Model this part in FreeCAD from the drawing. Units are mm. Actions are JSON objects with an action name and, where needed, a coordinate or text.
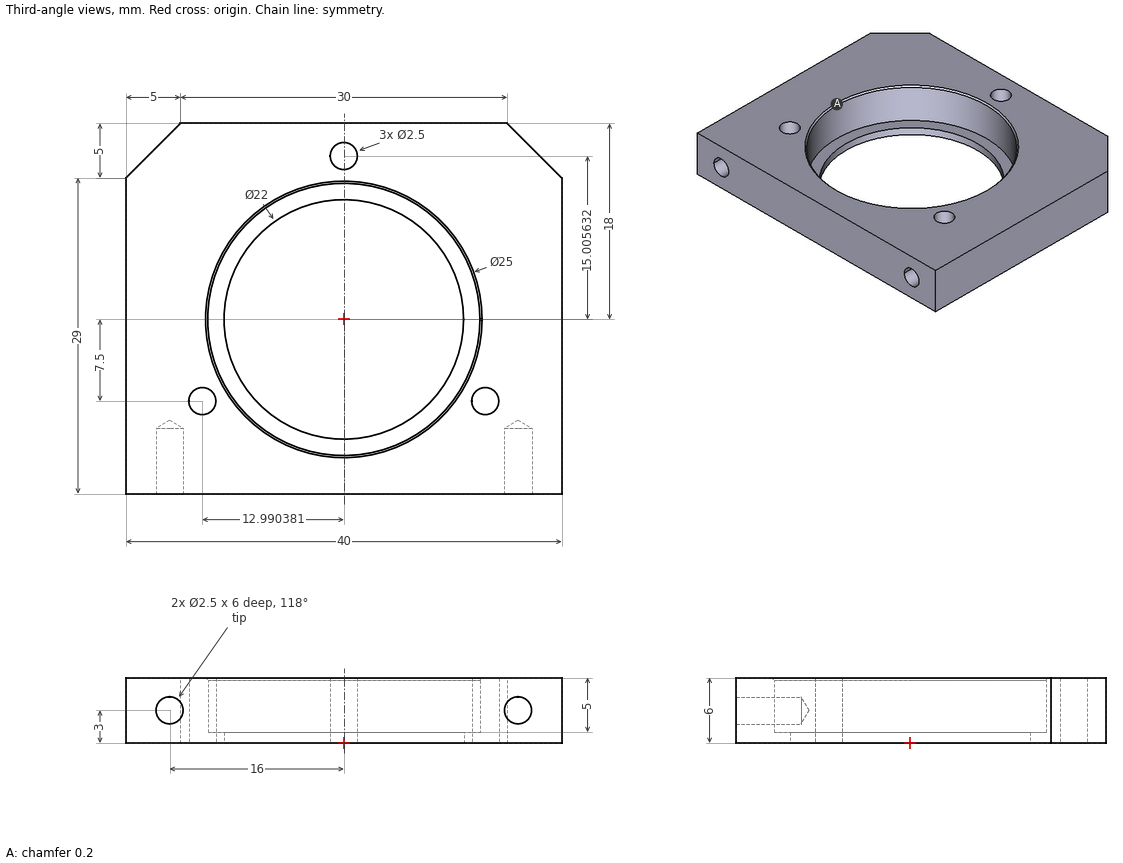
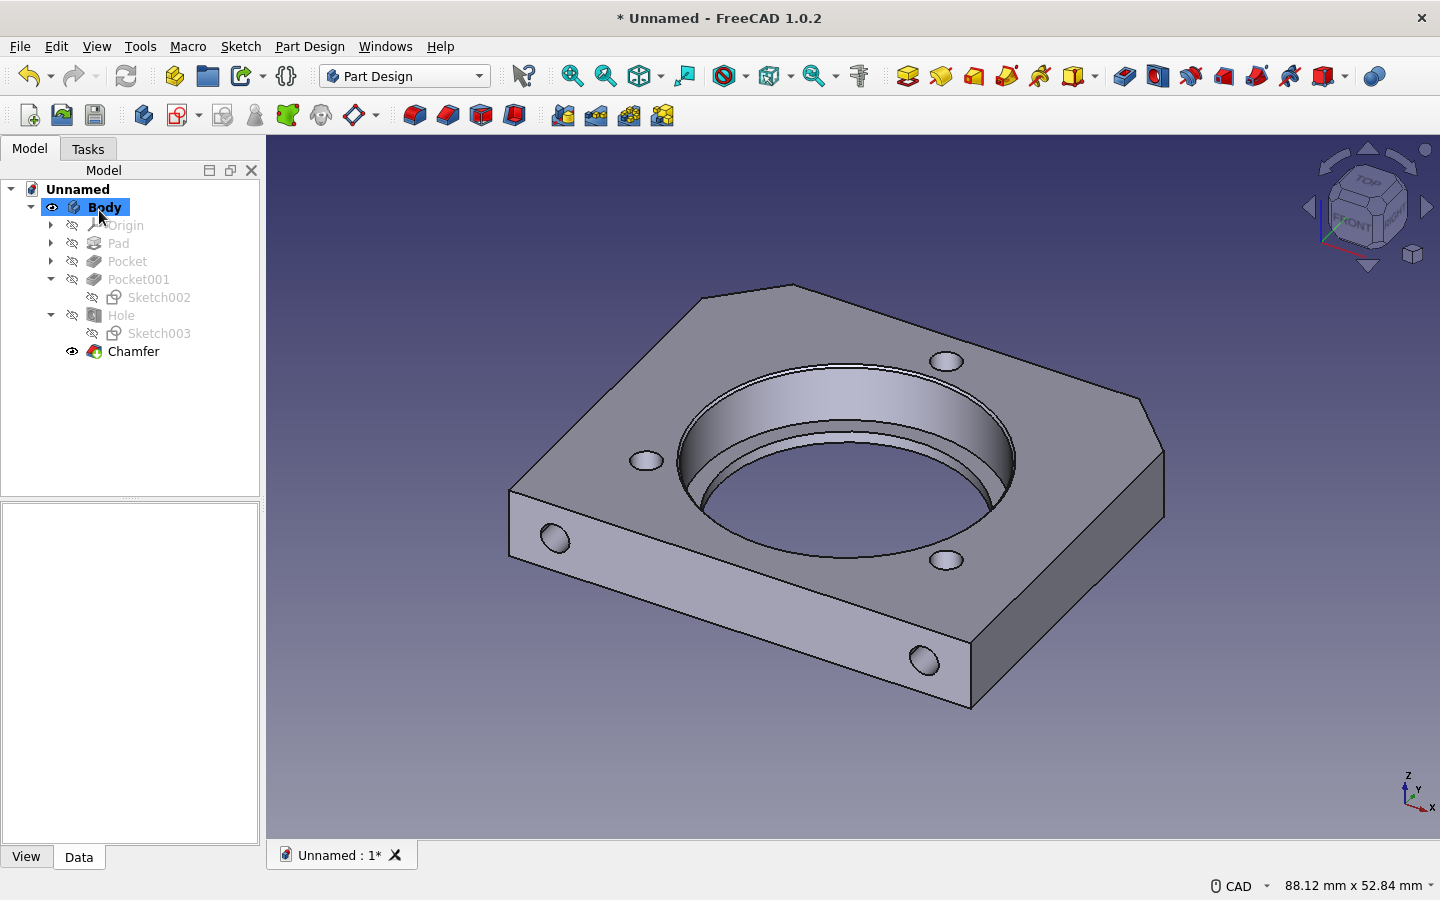
{"action": "key", "text": "0"}